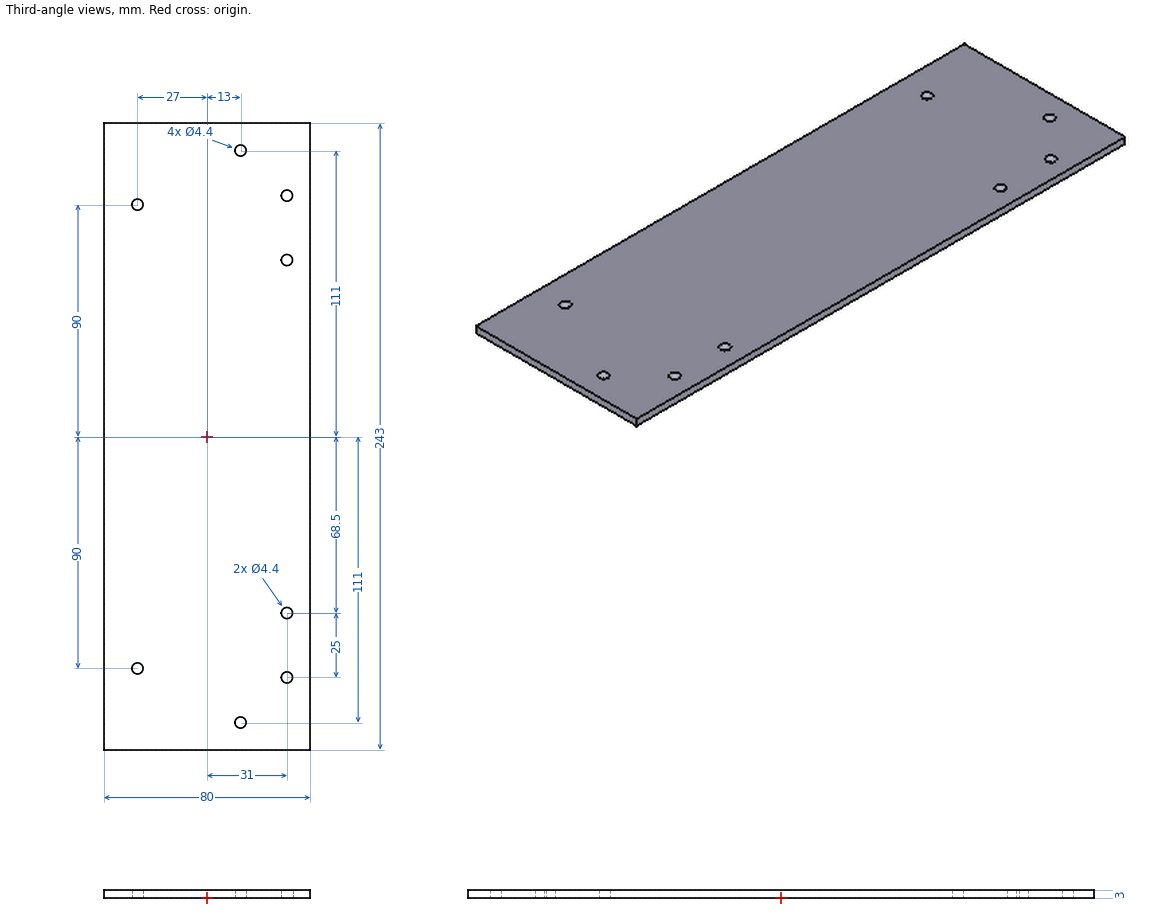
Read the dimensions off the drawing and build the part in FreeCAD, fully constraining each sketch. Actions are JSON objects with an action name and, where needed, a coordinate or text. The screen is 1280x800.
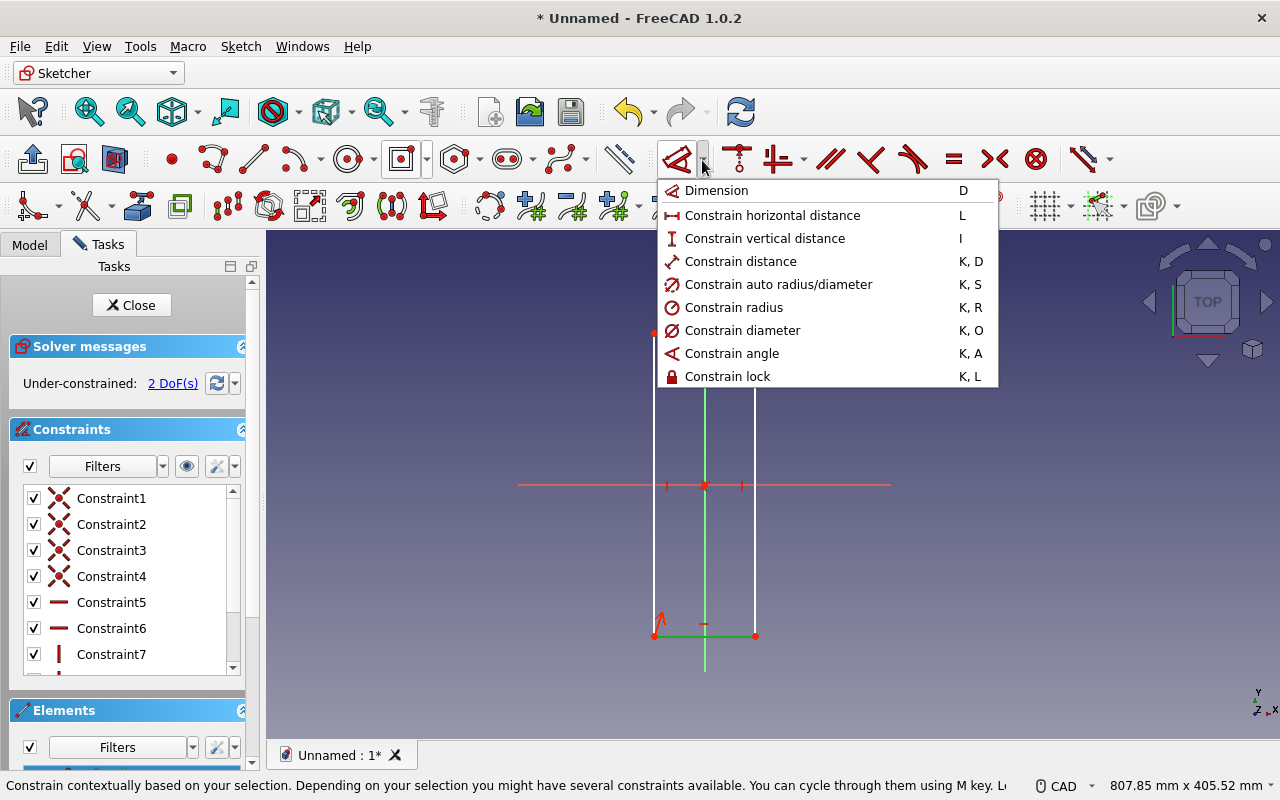
{"action": "left_click", "coordinate": [828, 216]}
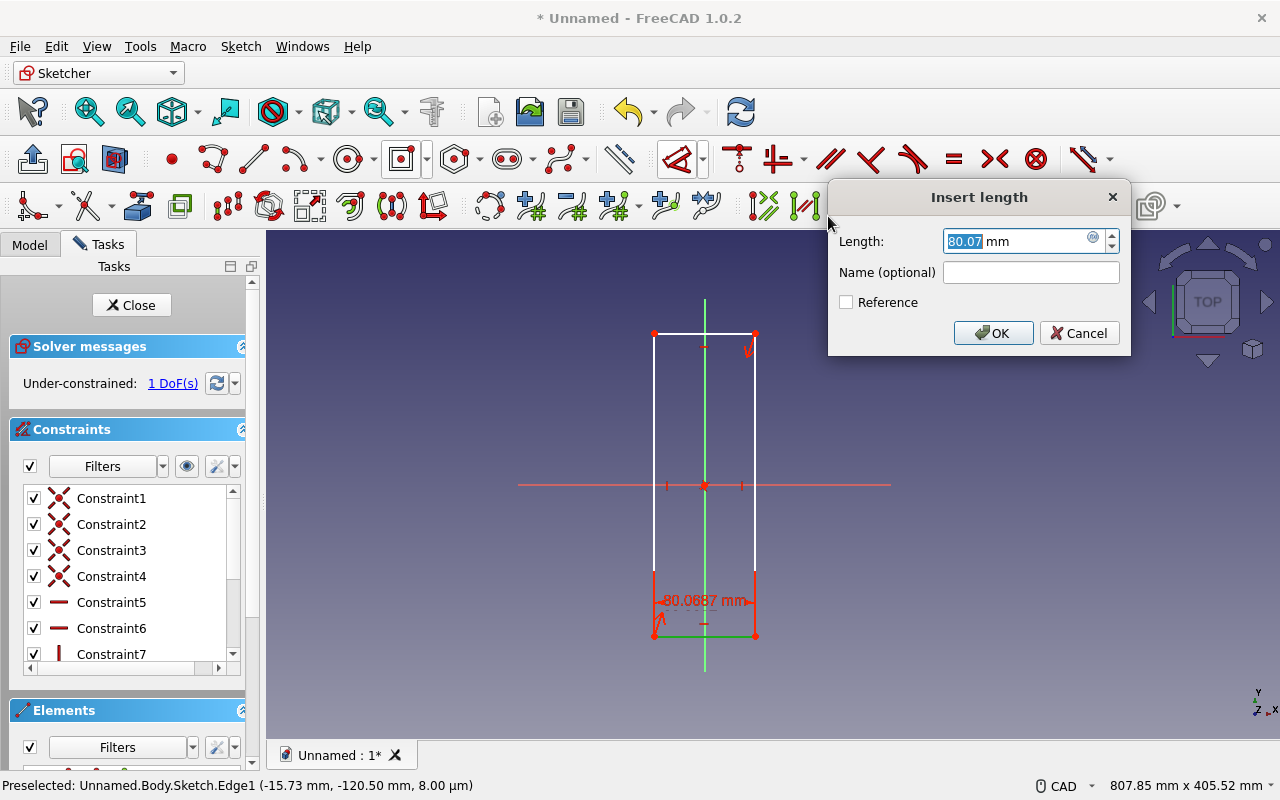
{"action": "type", "text": "80"}
{"action": "key", "text": "Return"}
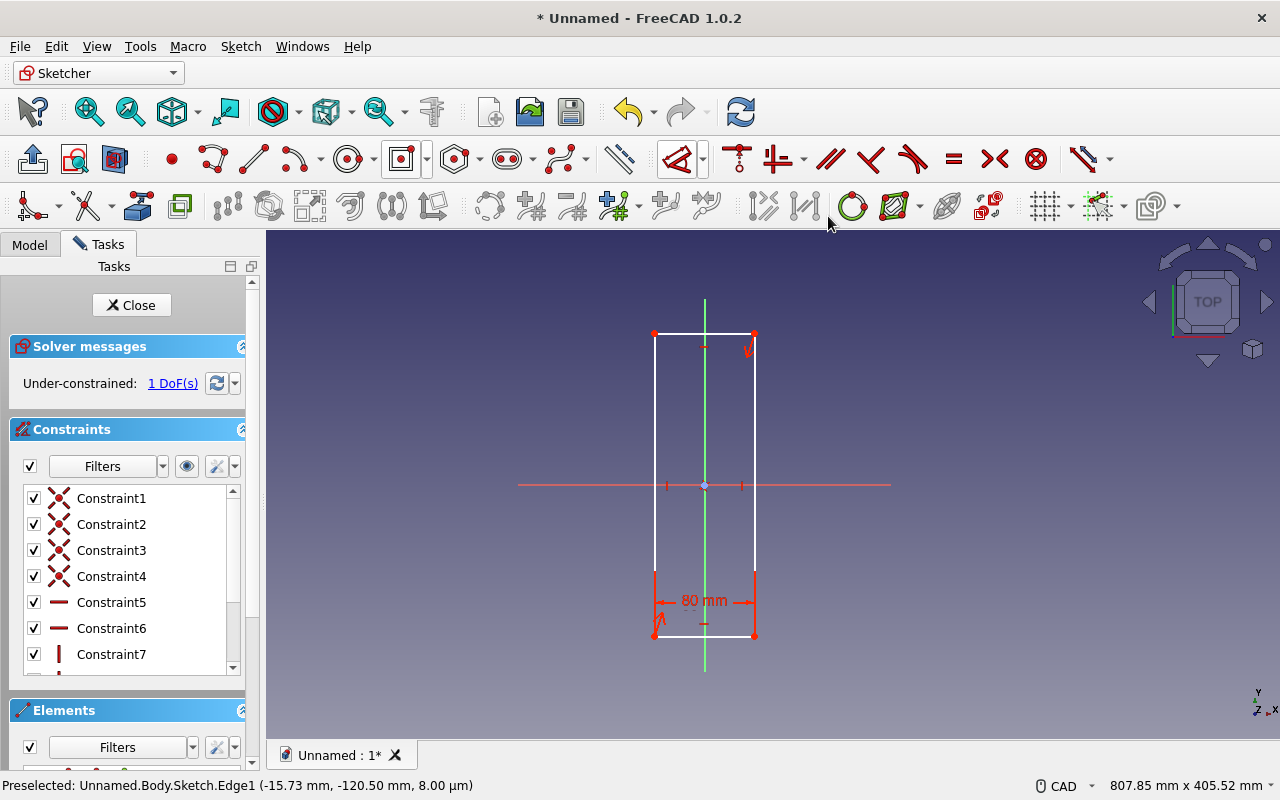
{"action": "left_click", "coordinate": [755, 546]}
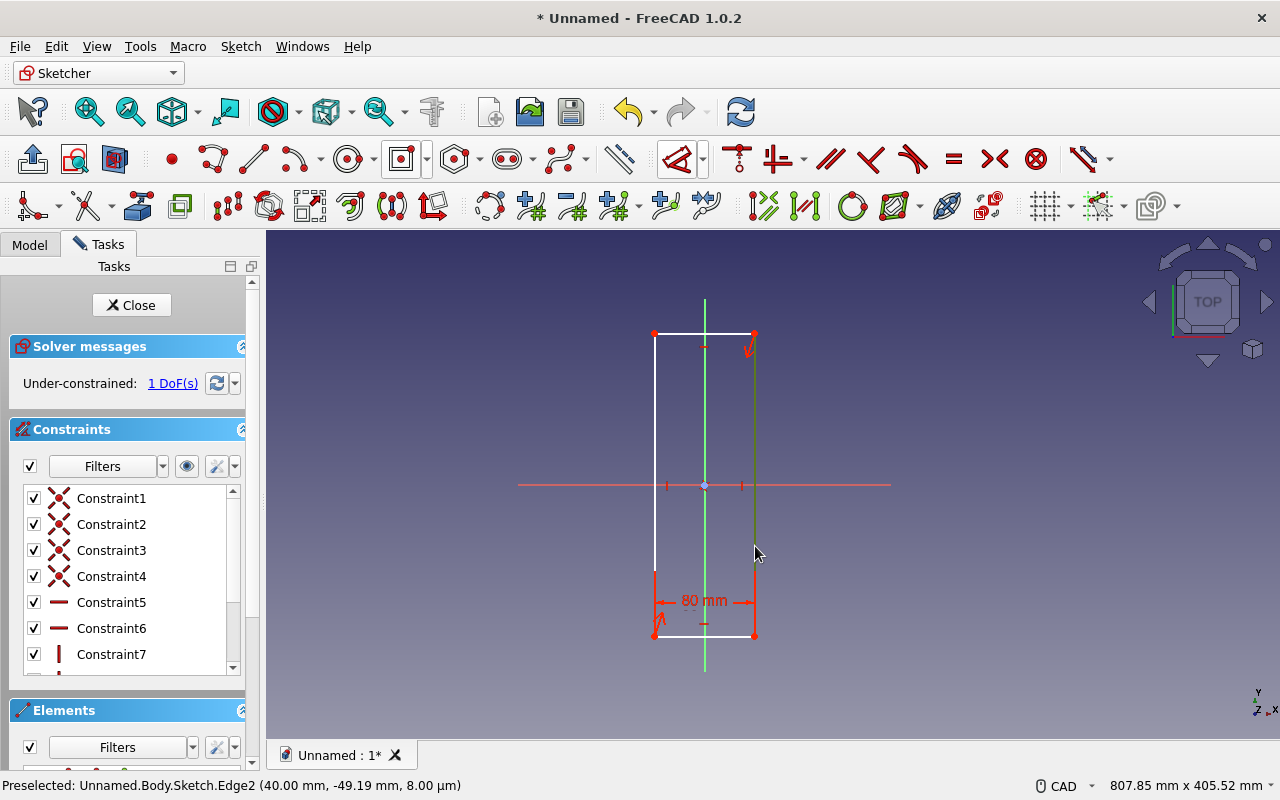
{"action": "key", "text": "i"}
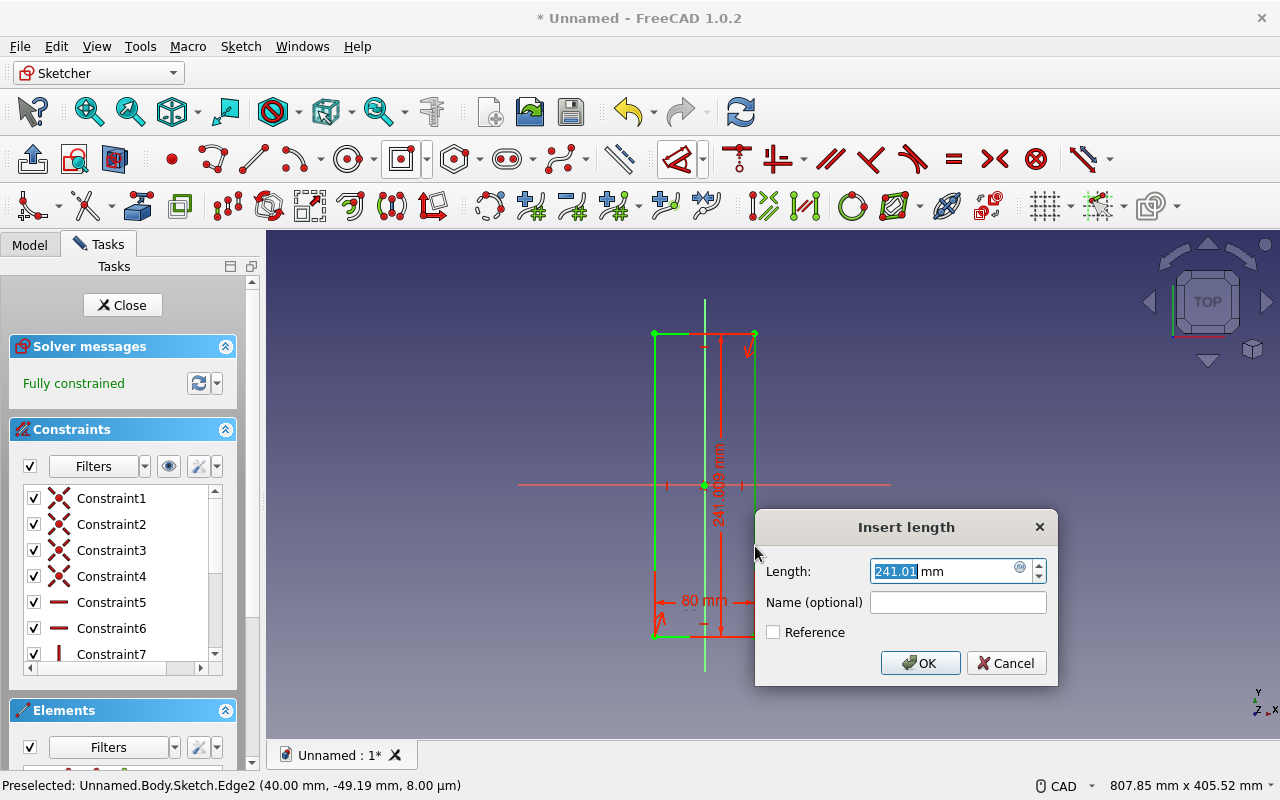
{"action": "type", "text": "243"}
{"action": "key", "text": "Return"}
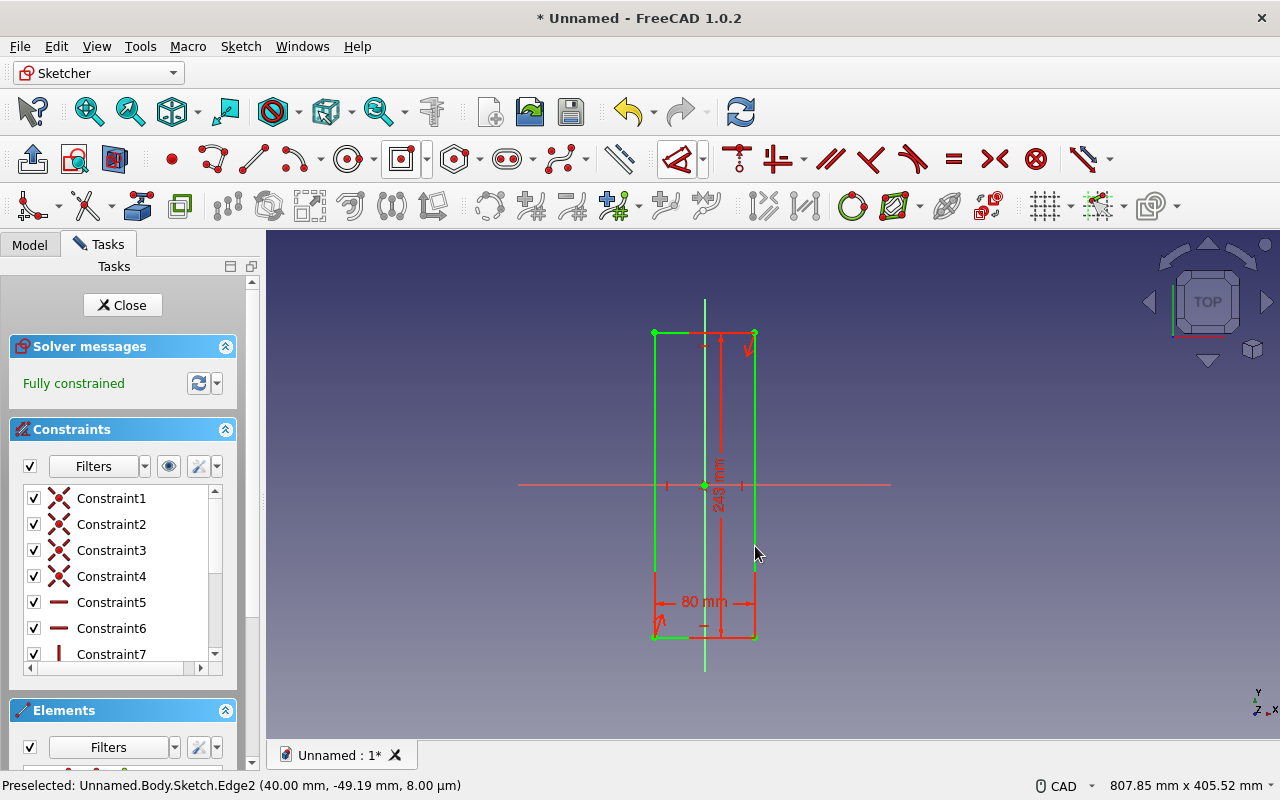
{"action": "left_click", "coordinate": [123, 305]}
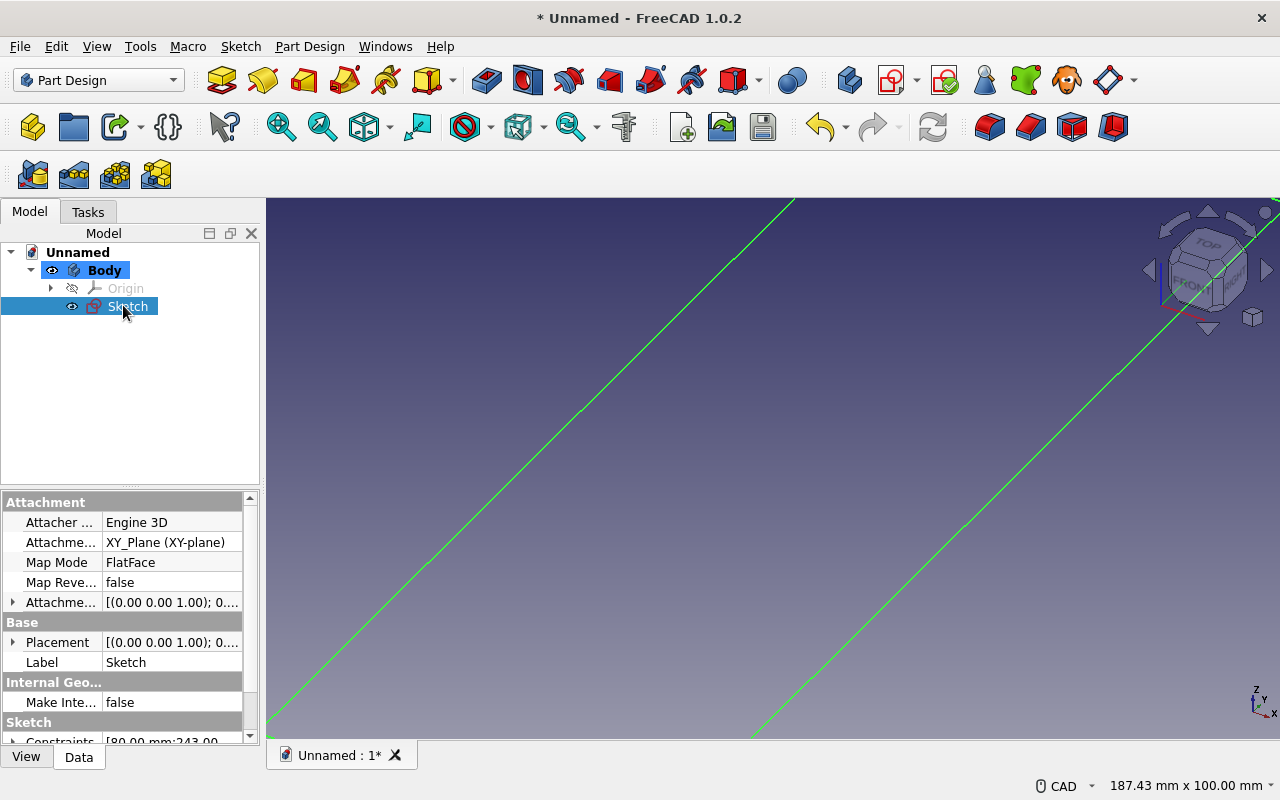
{"action": "left_click", "coordinate": [222, 80]}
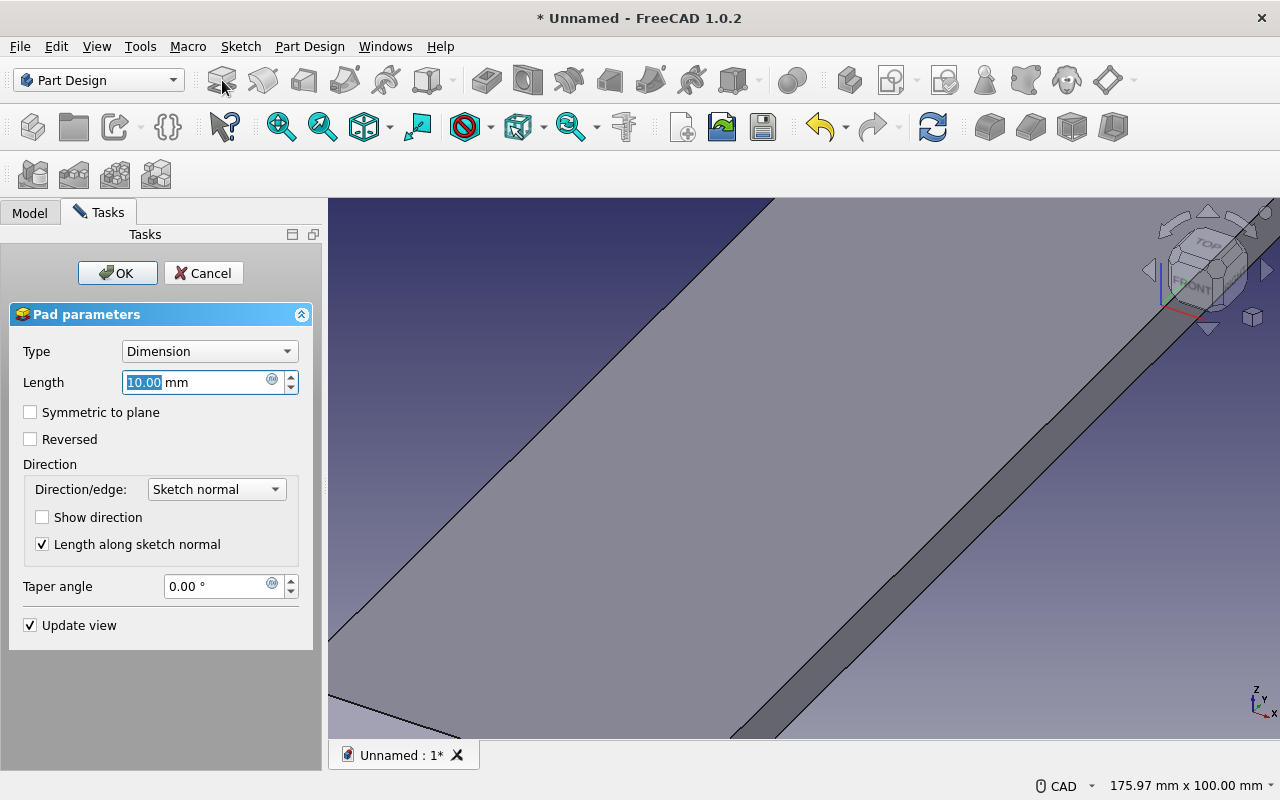
{"action": "type", "text": "3"}
{"action": "key", "text": "Tab"}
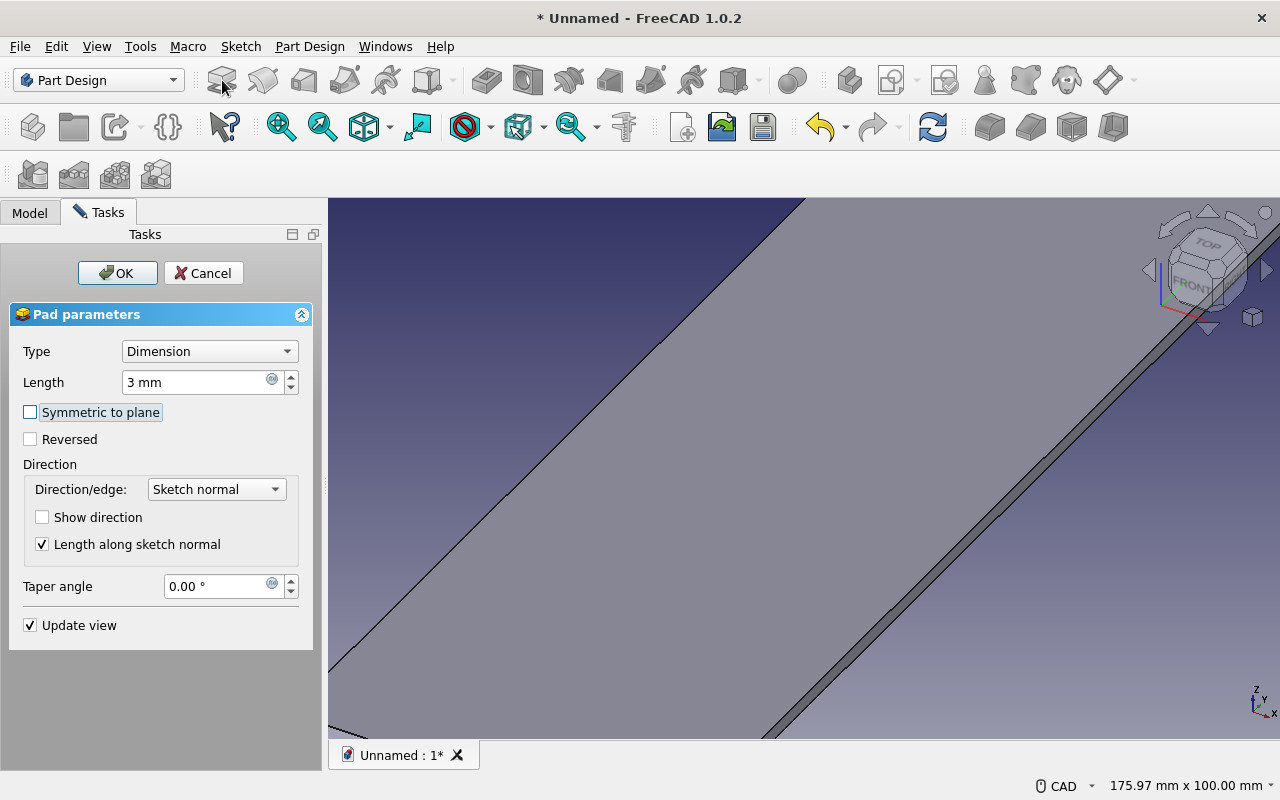
{"action": "left_click", "coordinate": [118, 273]}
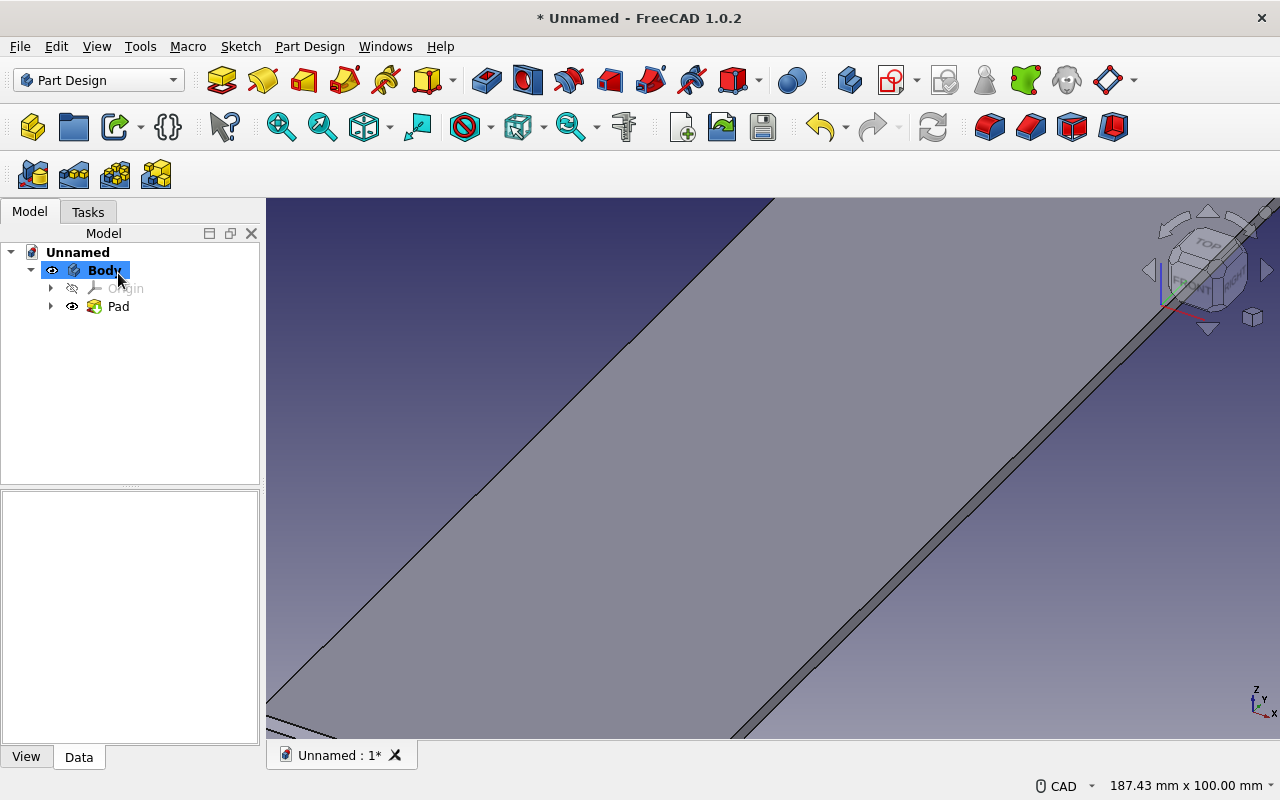
{"action": "left_click", "coordinate": [282, 128]}